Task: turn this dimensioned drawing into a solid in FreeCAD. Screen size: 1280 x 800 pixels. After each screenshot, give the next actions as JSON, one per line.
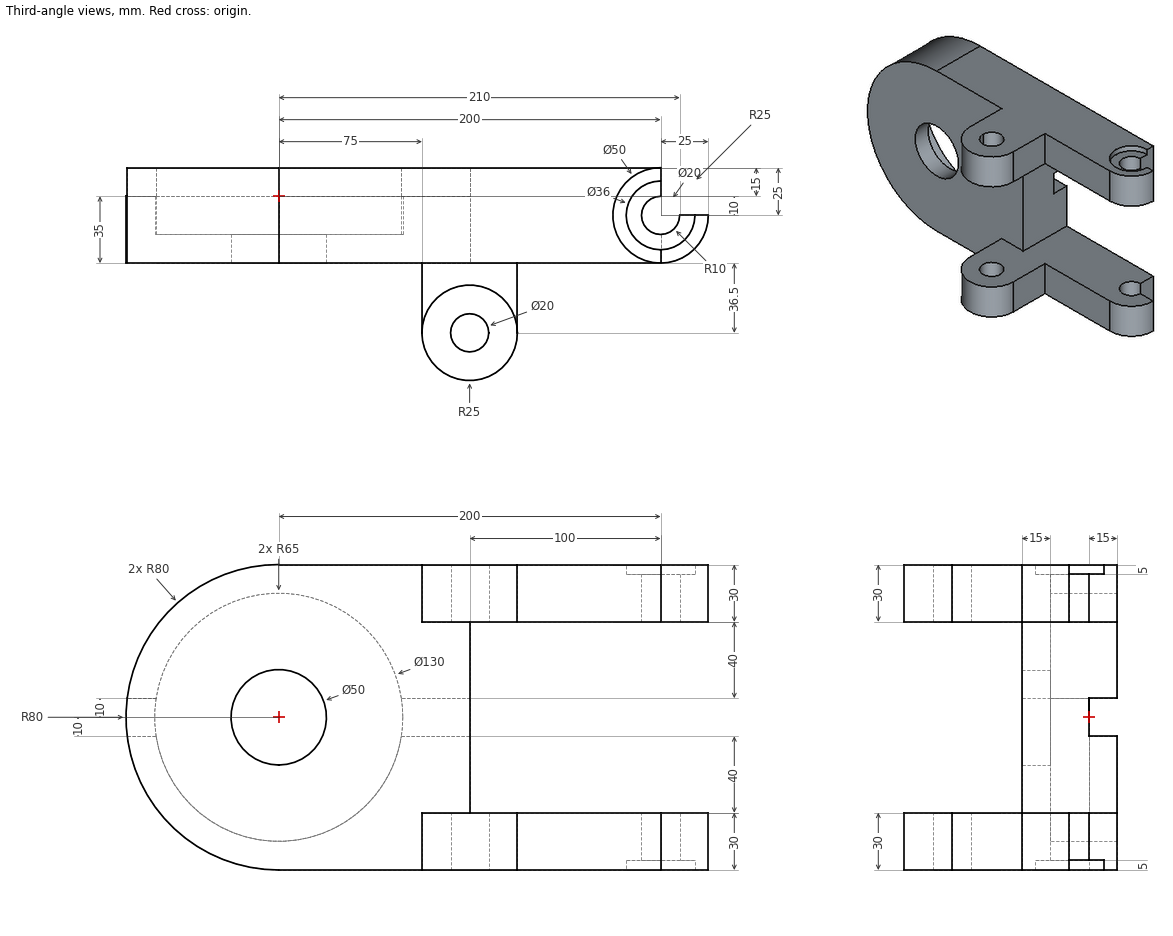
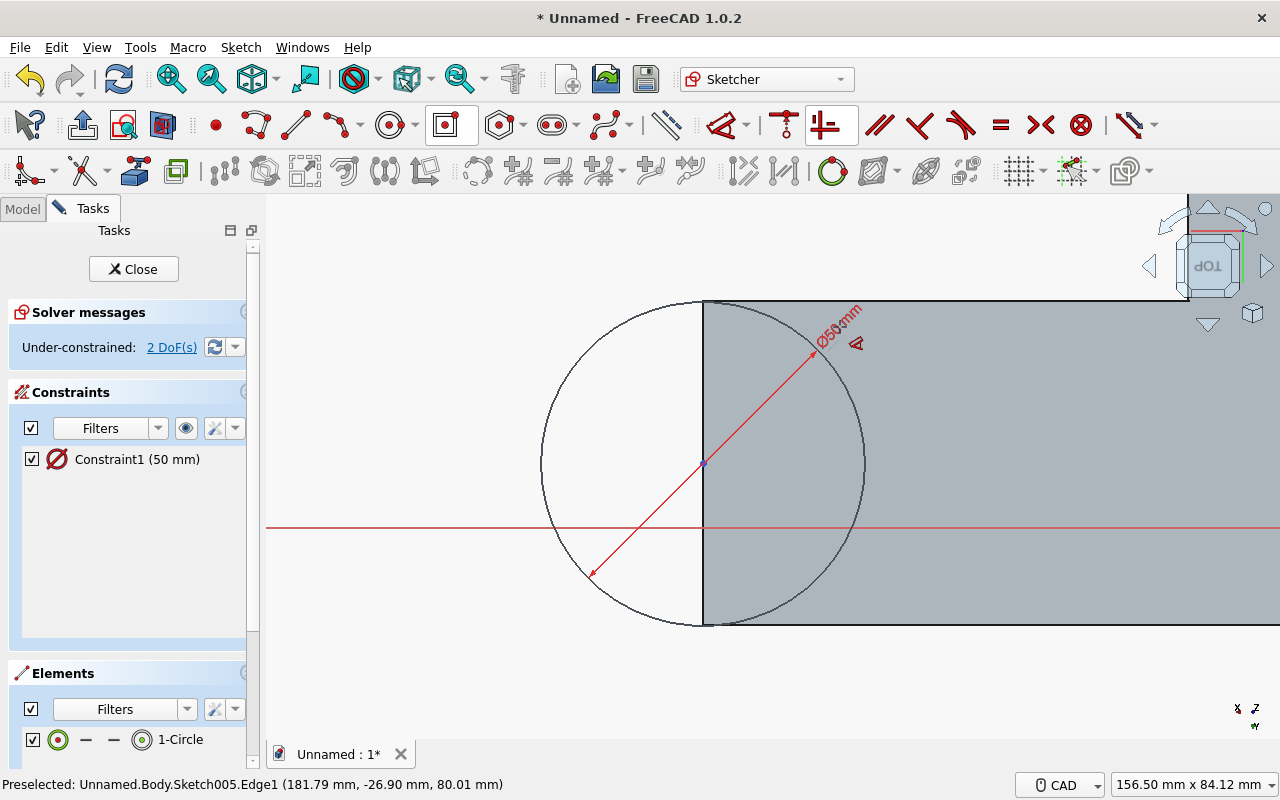
{"action": "left_click", "coordinate": [703, 464]}
{"action": "left_click", "coordinate": [669, 496]}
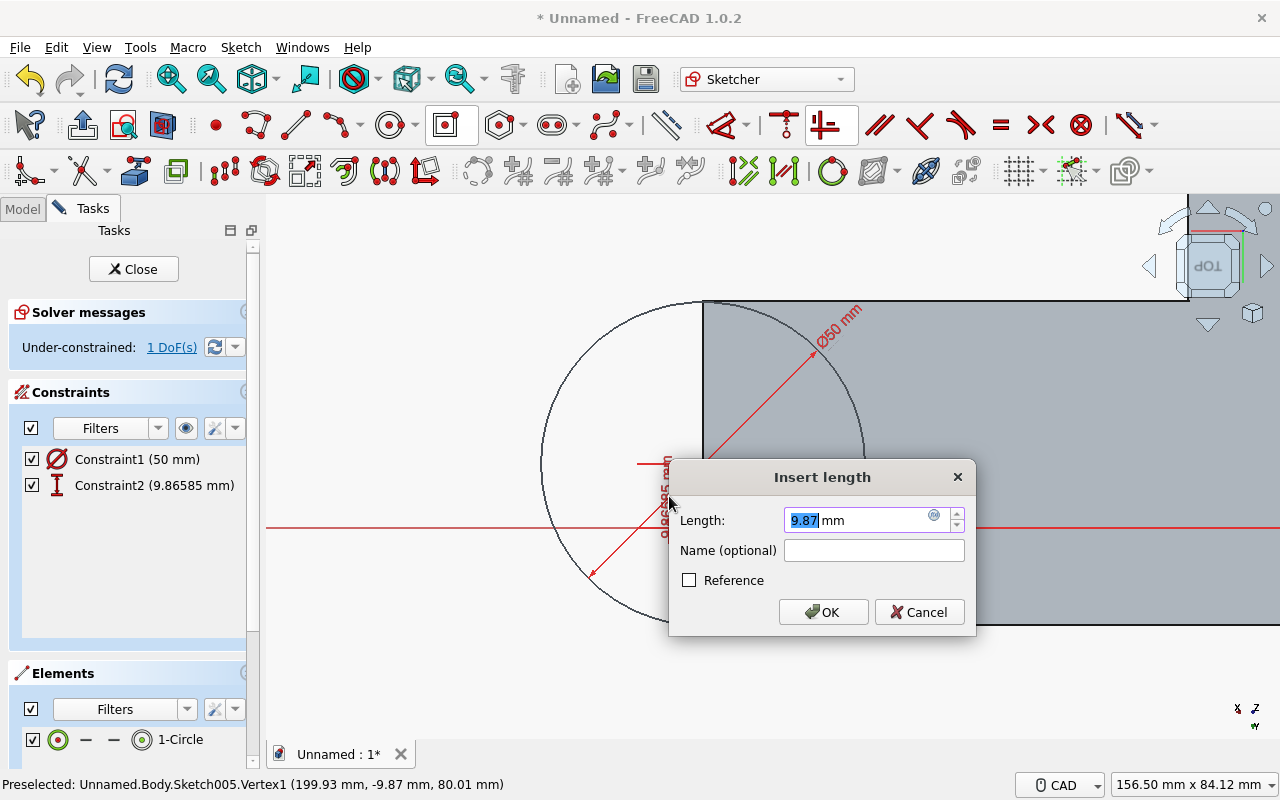
{"action": "type", "text": "10"}
{"action": "key", "text": "Return"}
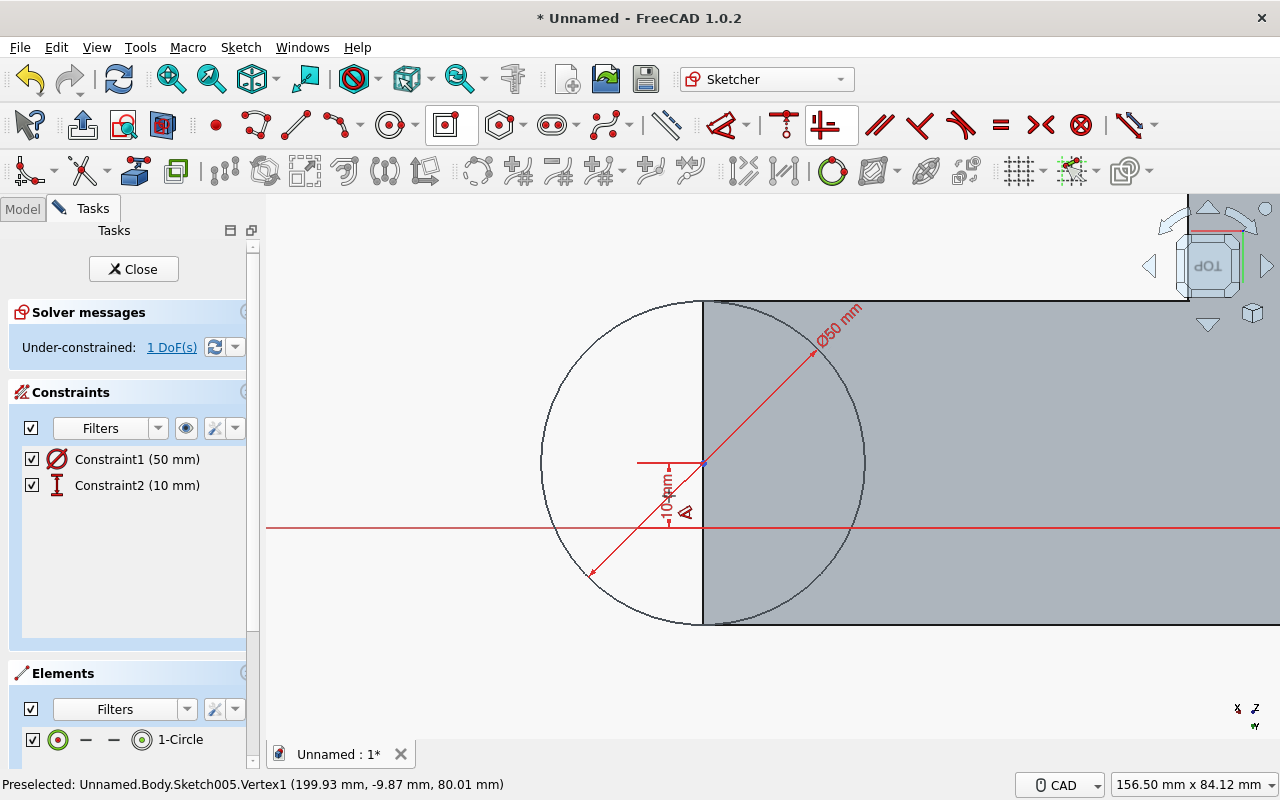
{"action": "left_click", "coordinate": [703, 463]}
{"action": "left_click", "coordinate": [909, 562]}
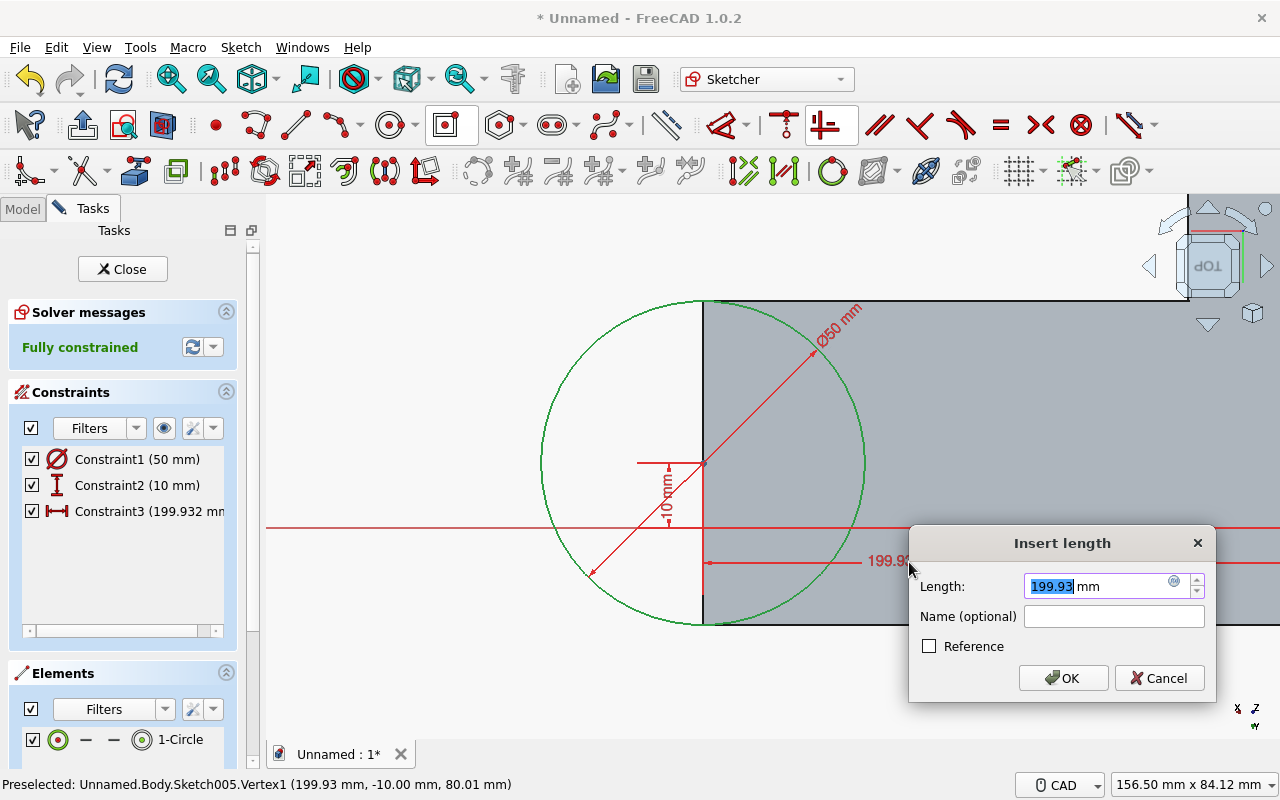
{"action": "type", "text": "200"}
{"action": "key", "text": "Return"}
{"action": "key", "text": "Escape"}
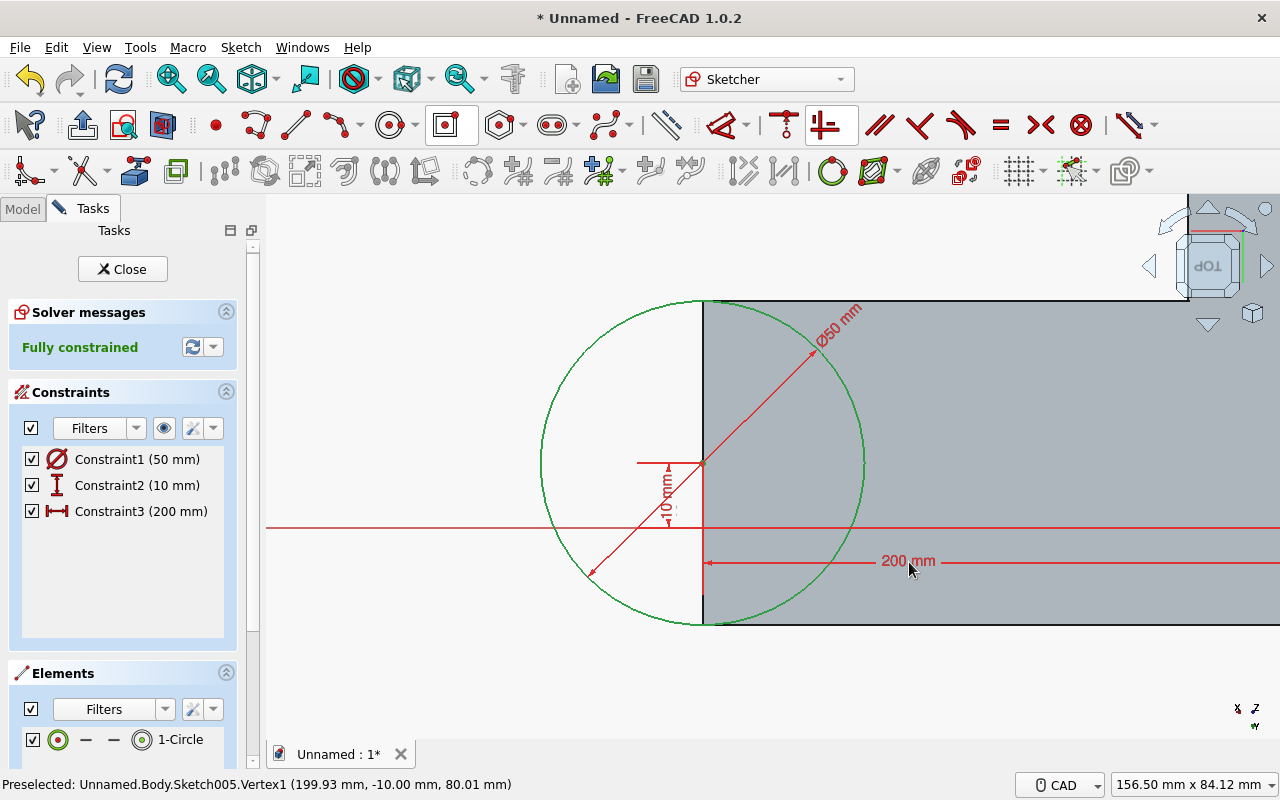
{"action": "left_click", "coordinate": [123, 269]}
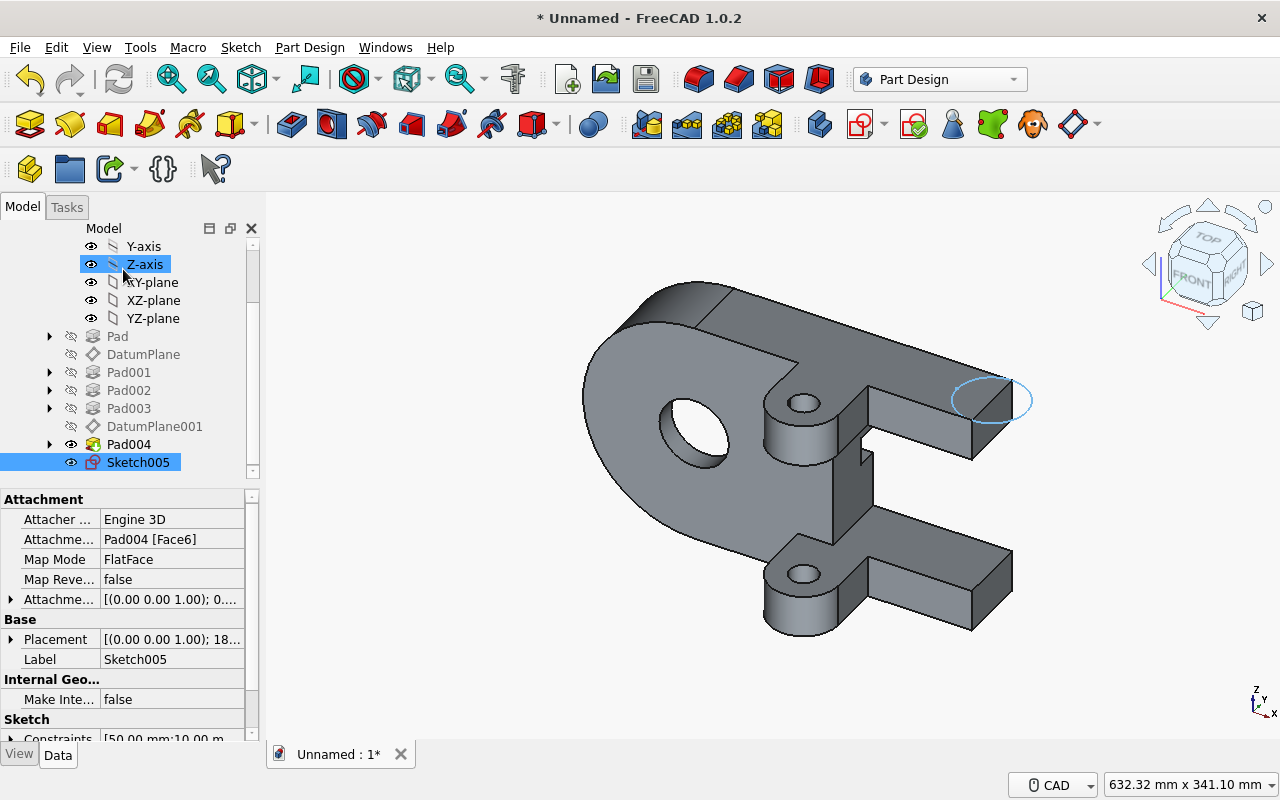
{"action": "left_click", "coordinate": [30, 124]}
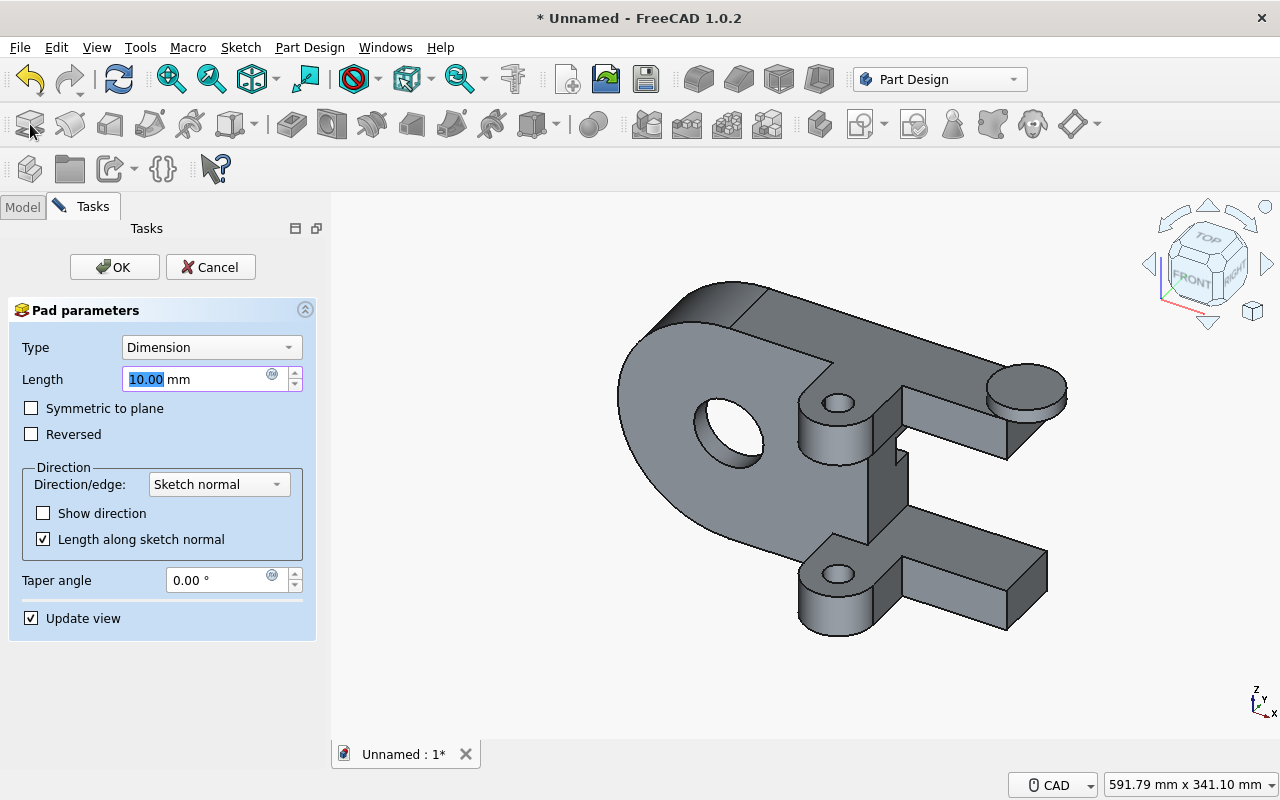
{"action": "type", "text": "30"}
{"action": "key", "text": "Tab"}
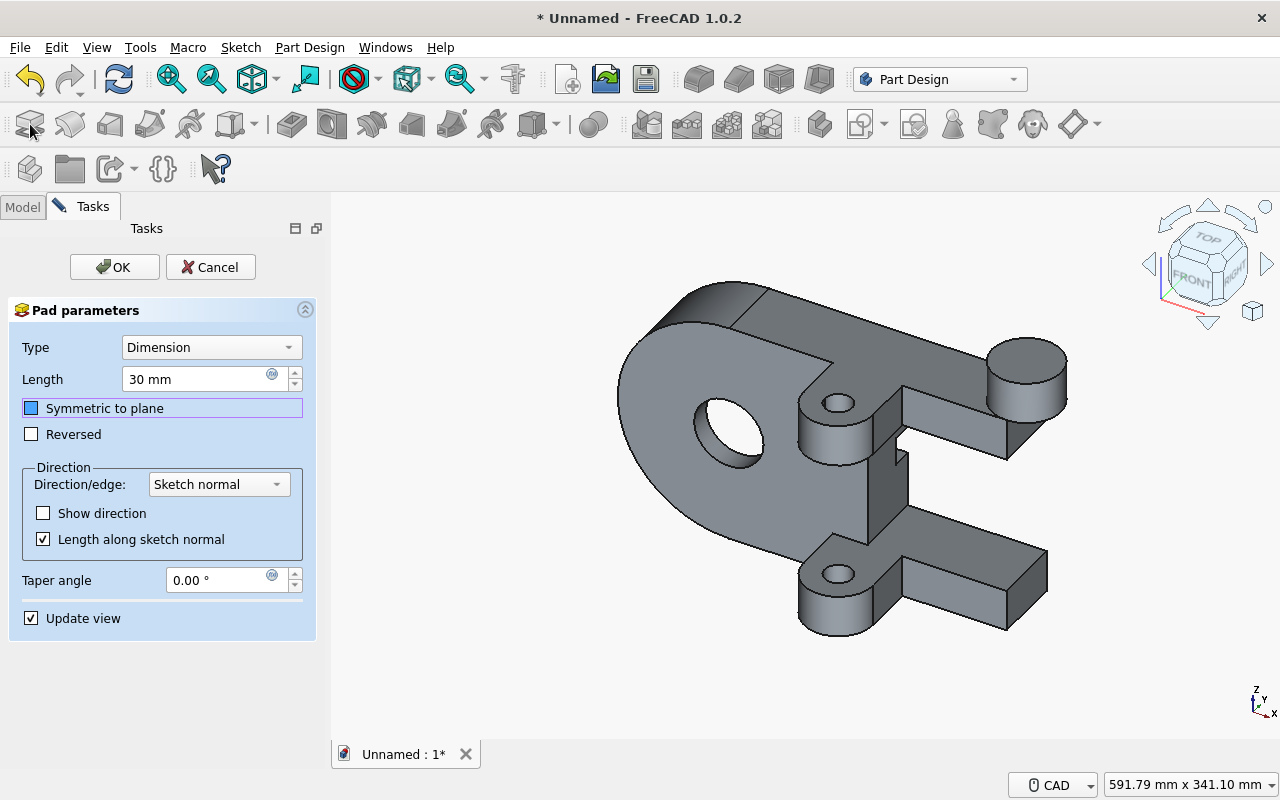
{"action": "left_click", "coordinate": [30, 434]}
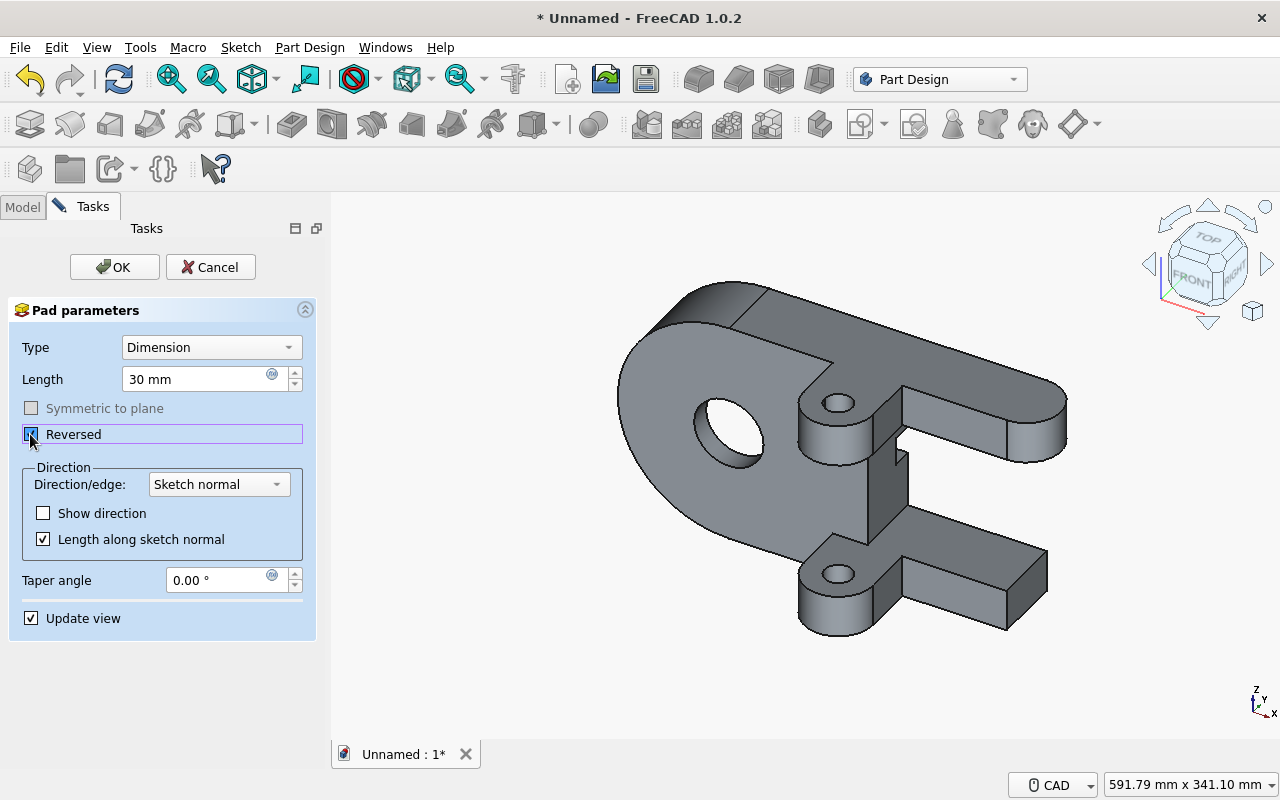
{"action": "left_click", "coordinate": [115, 267]}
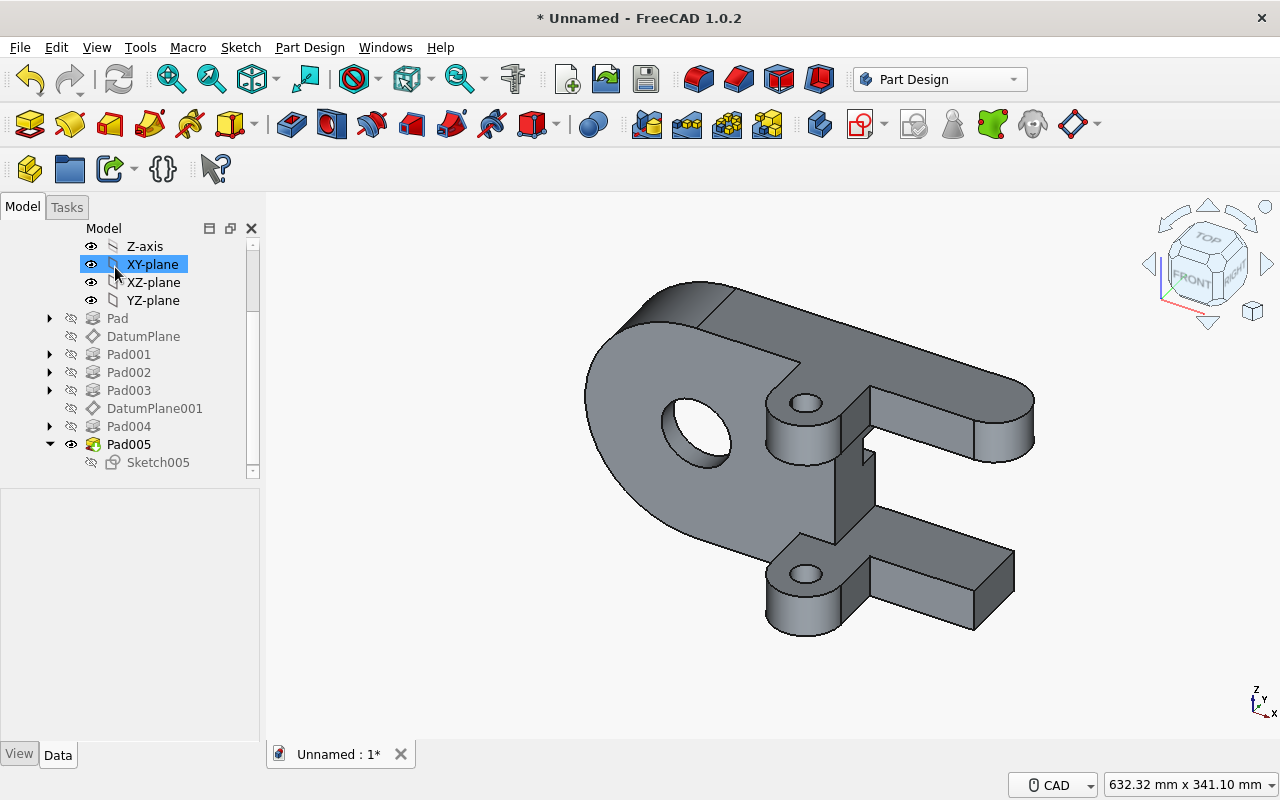
{"action": "left_click", "coordinate": [963, 388]}